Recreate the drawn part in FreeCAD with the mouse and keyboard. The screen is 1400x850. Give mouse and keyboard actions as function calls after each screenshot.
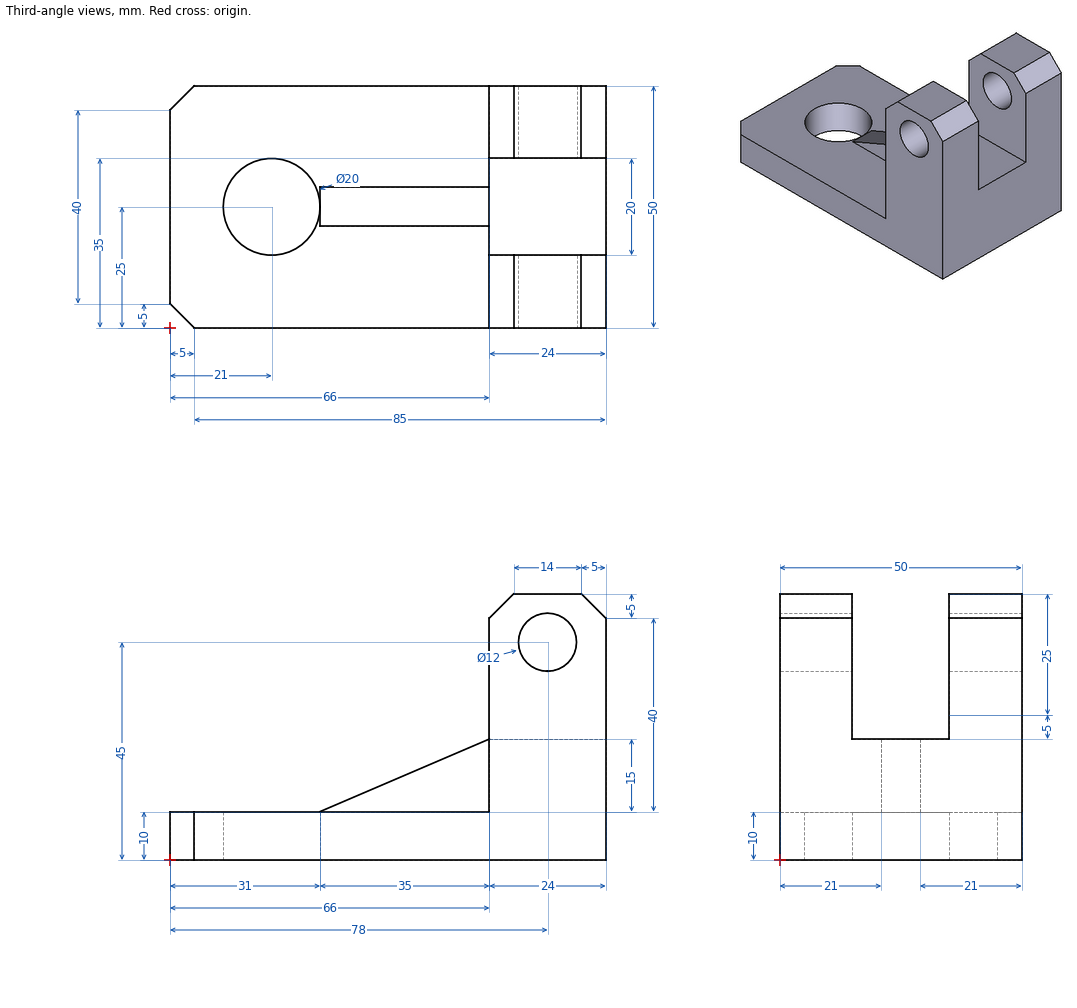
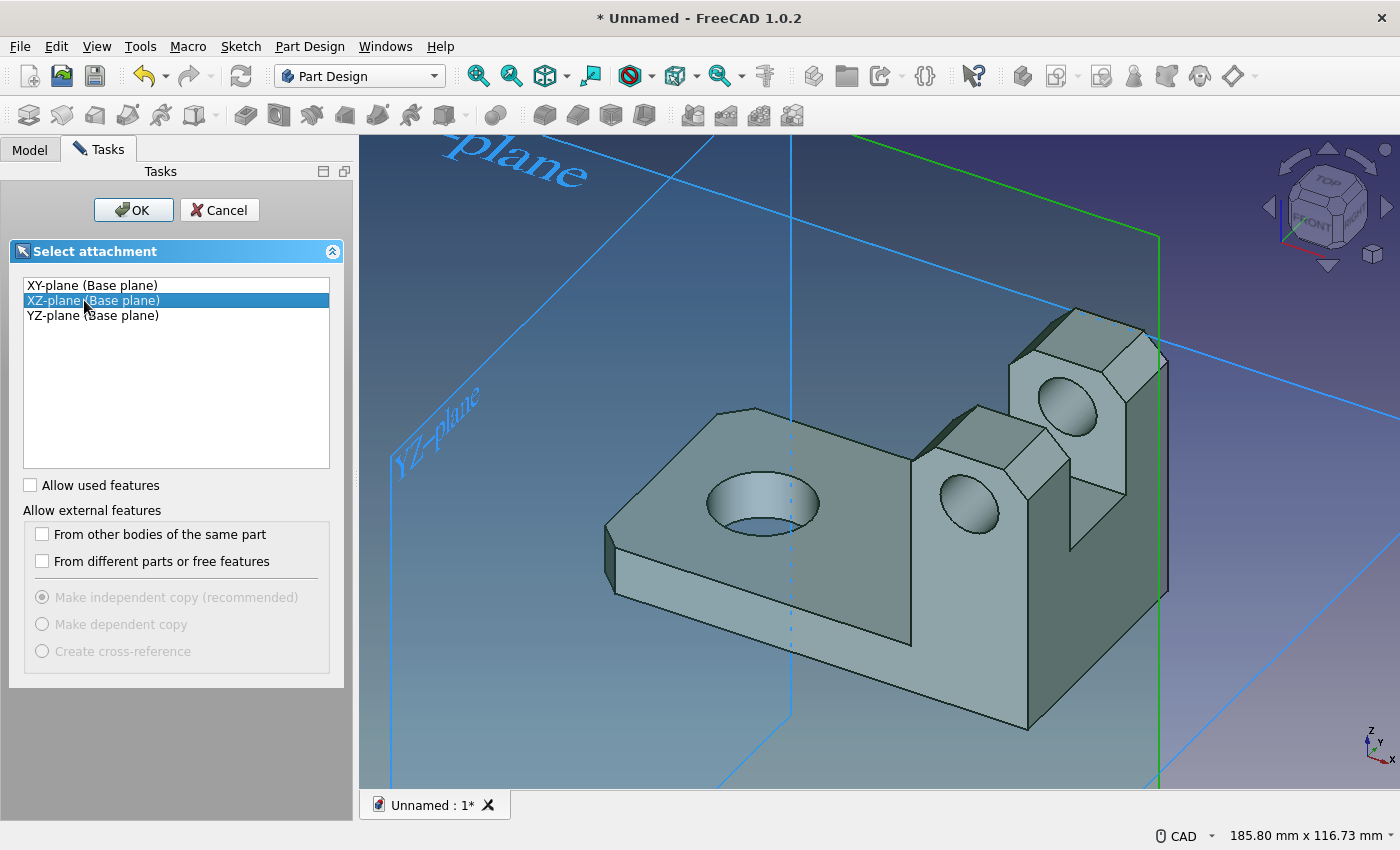
click(134, 210)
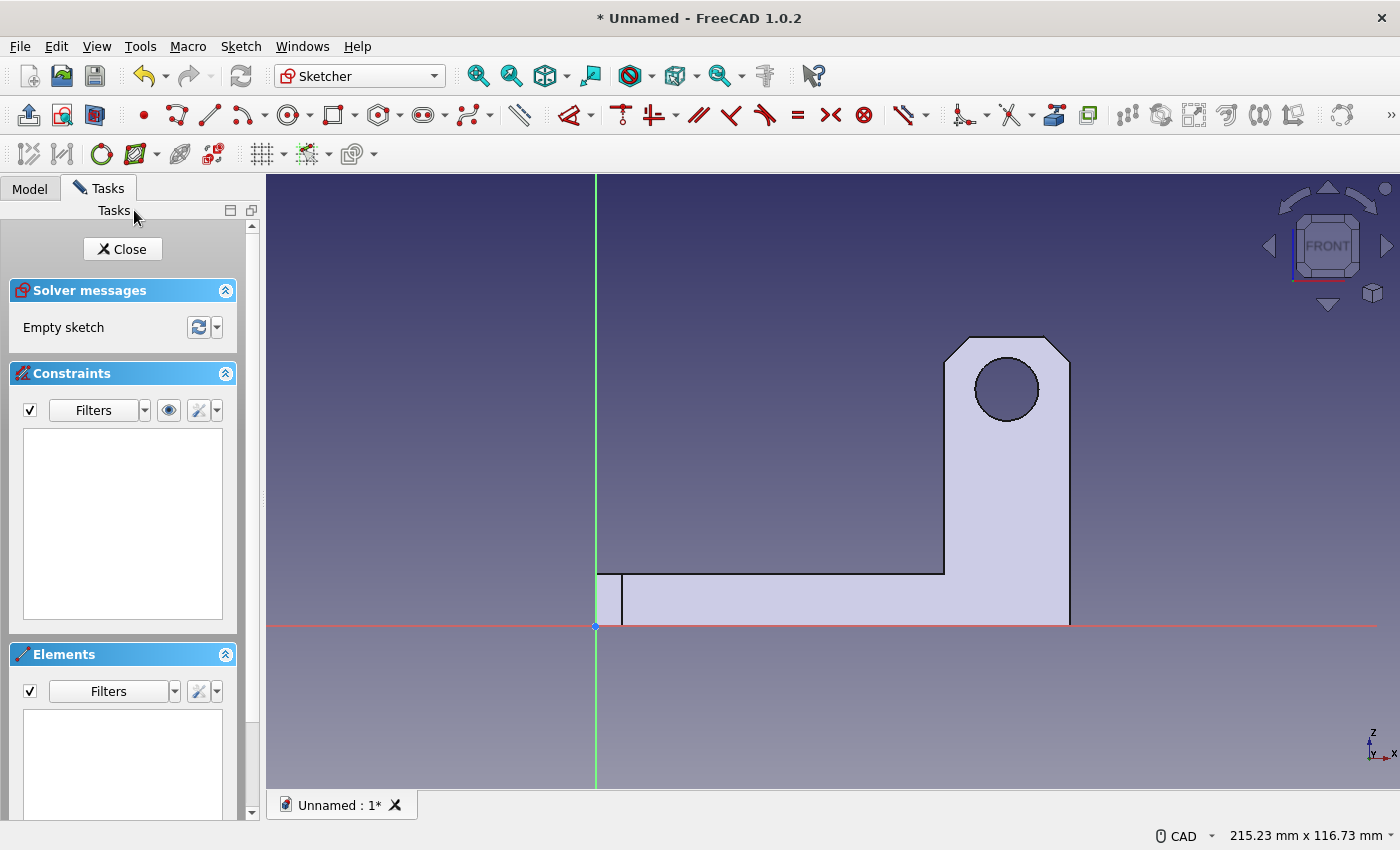
scroll(776, 657, up, 3)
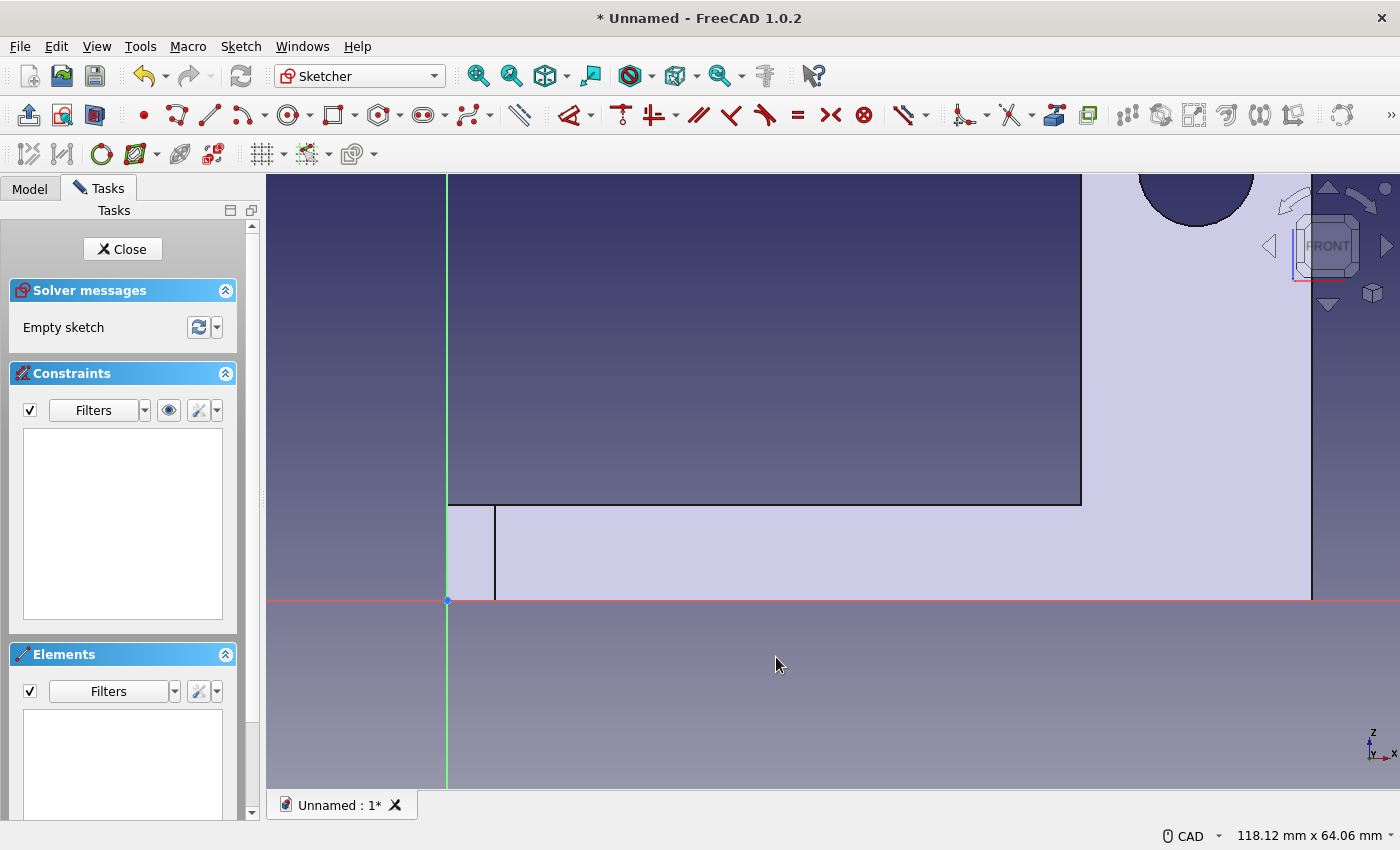
click(177, 116)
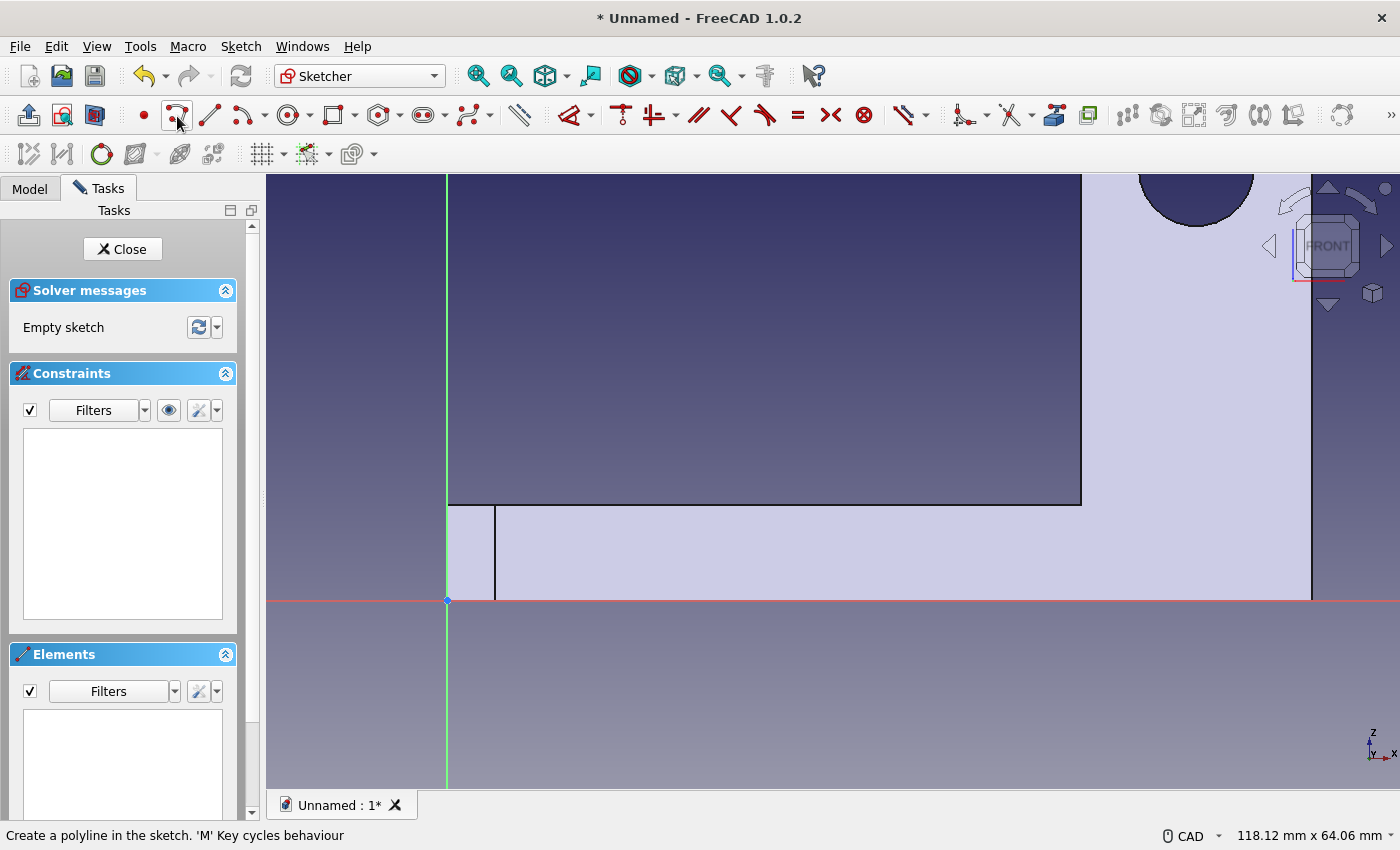
click(745, 505)
click(1081, 505)
click(1081, 361)
click(745, 506)
key(Escape)
key(Escape)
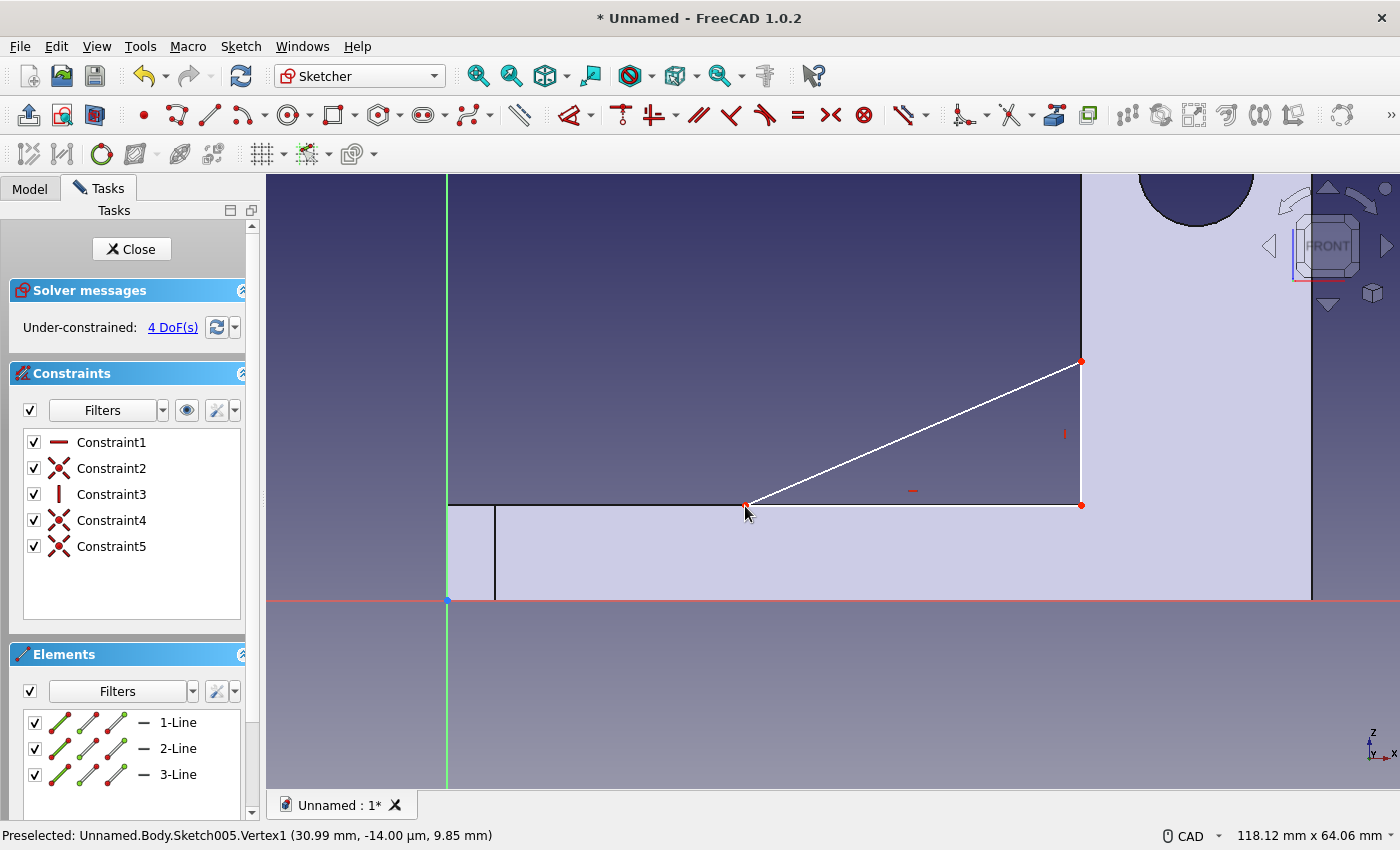
click(568, 116)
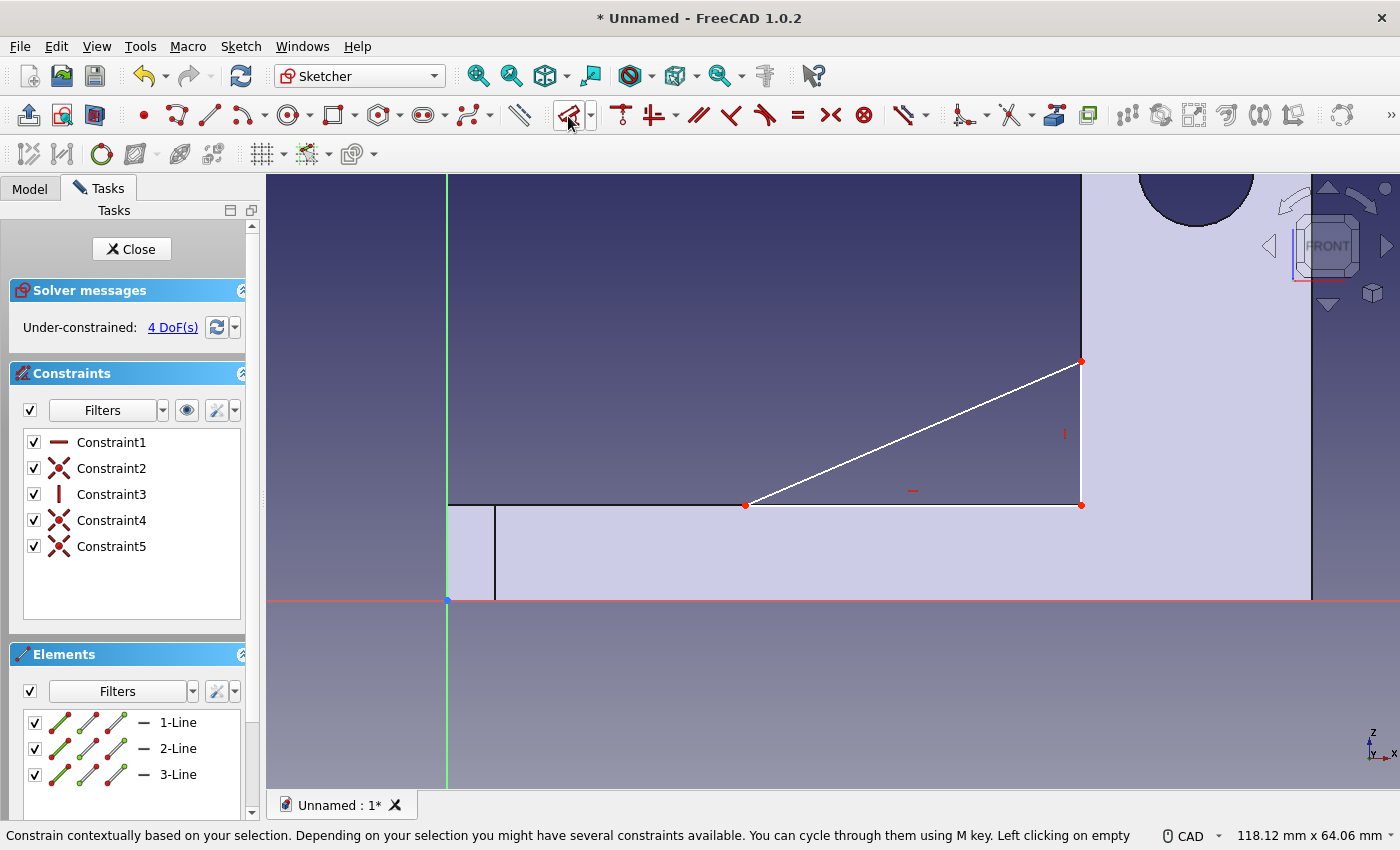
click(846, 506)
click(913, 540)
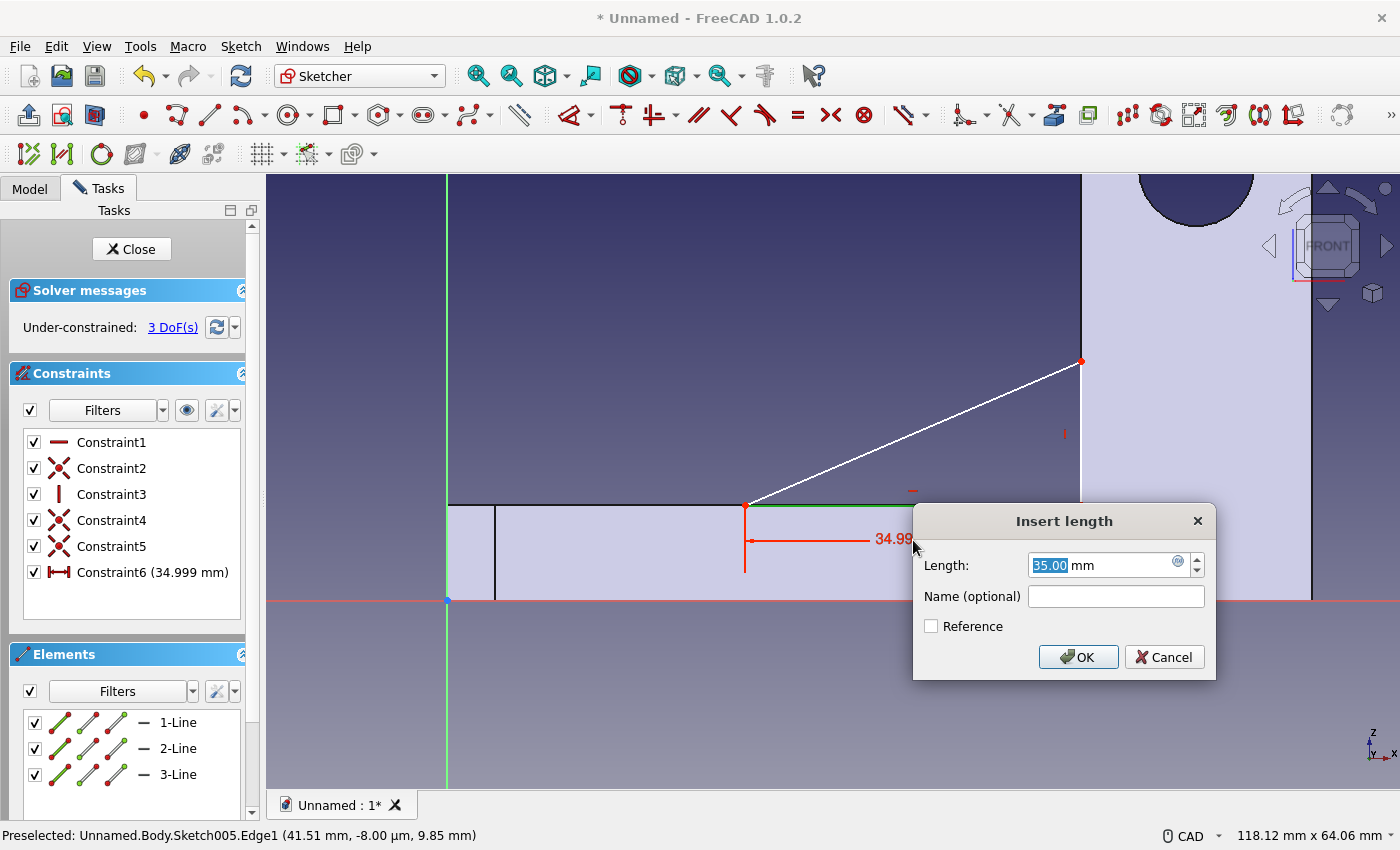
text(35)
key(Return)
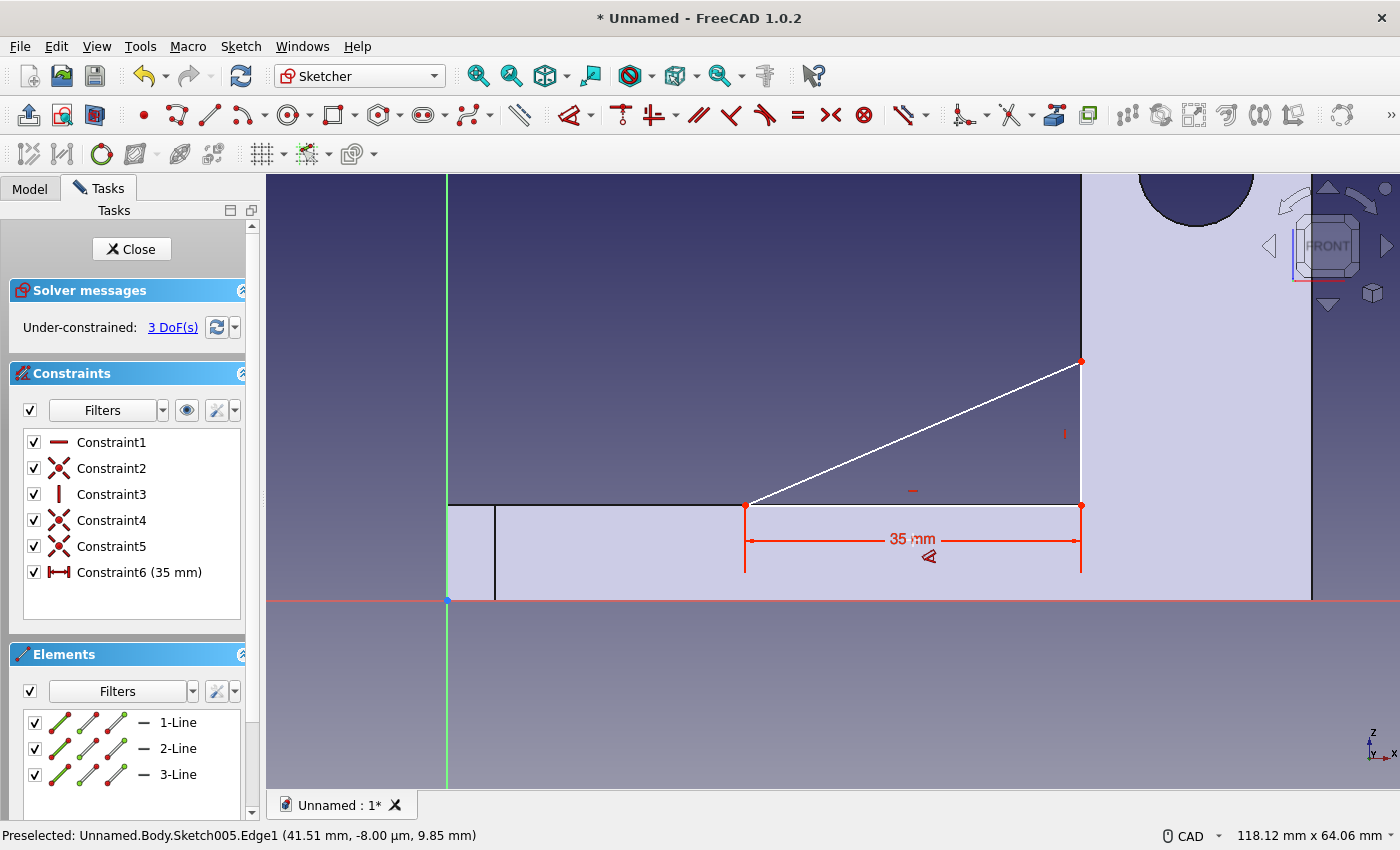
click(1081, 463)
click(1115, 434)